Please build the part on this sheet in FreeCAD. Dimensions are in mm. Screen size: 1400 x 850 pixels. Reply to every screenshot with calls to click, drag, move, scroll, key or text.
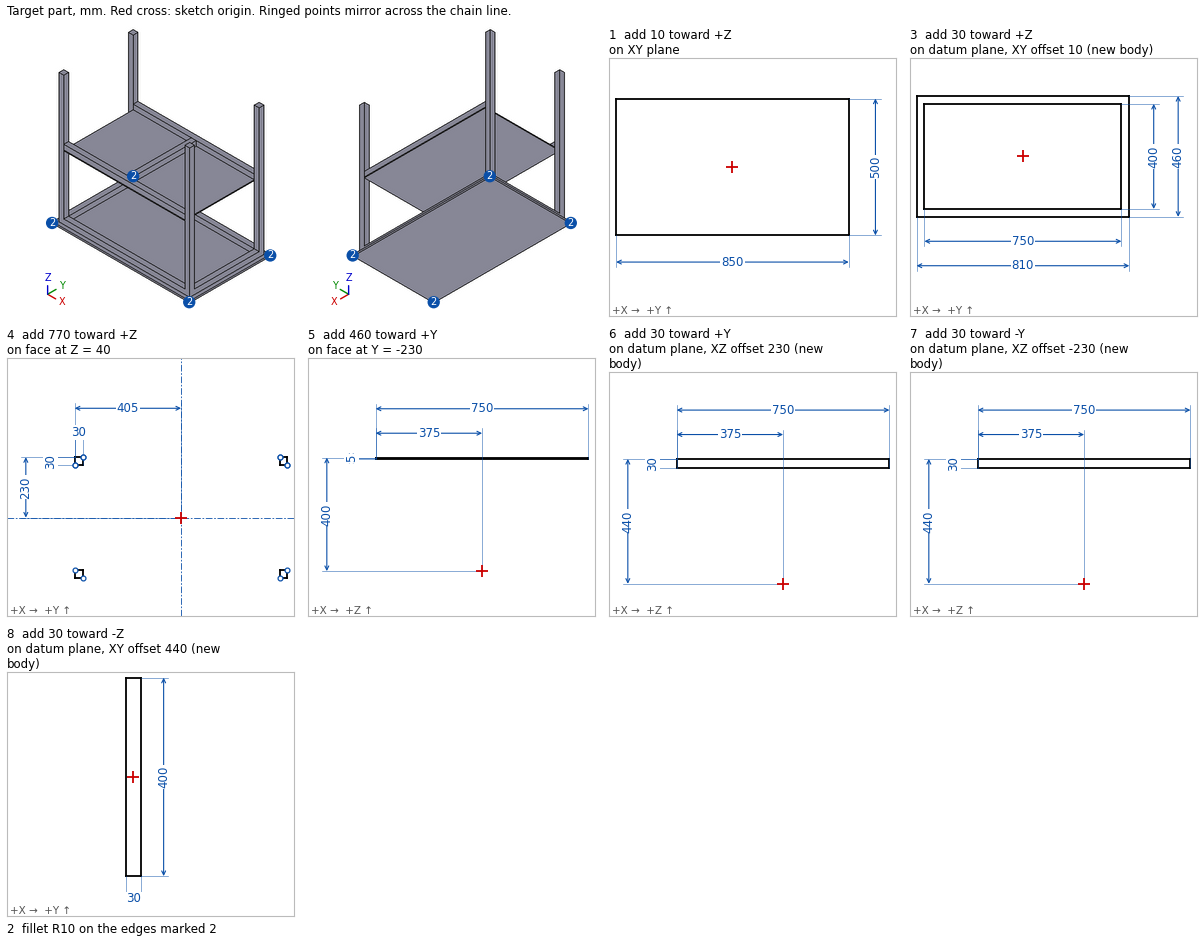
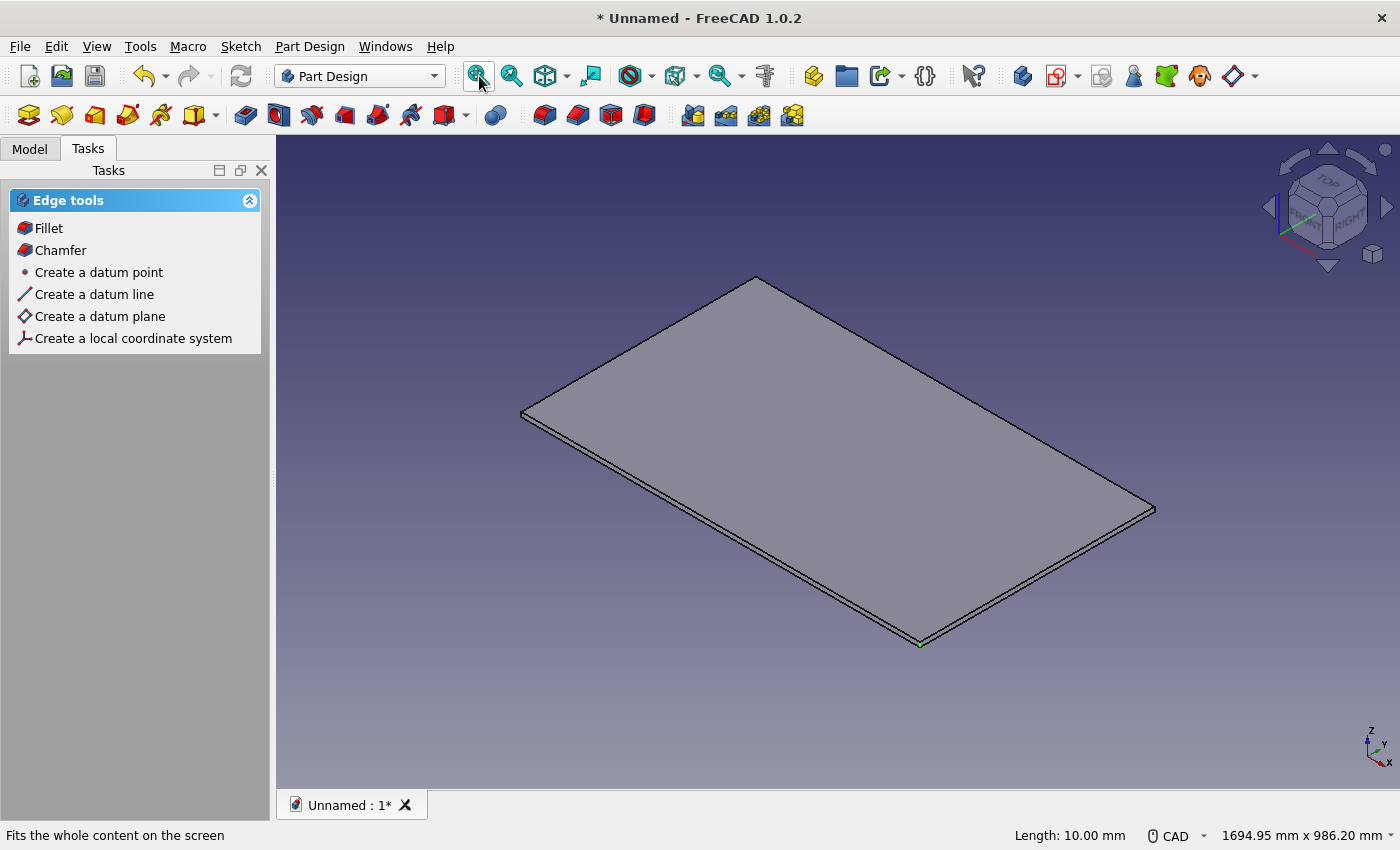
scroll(521, 414, up, 9)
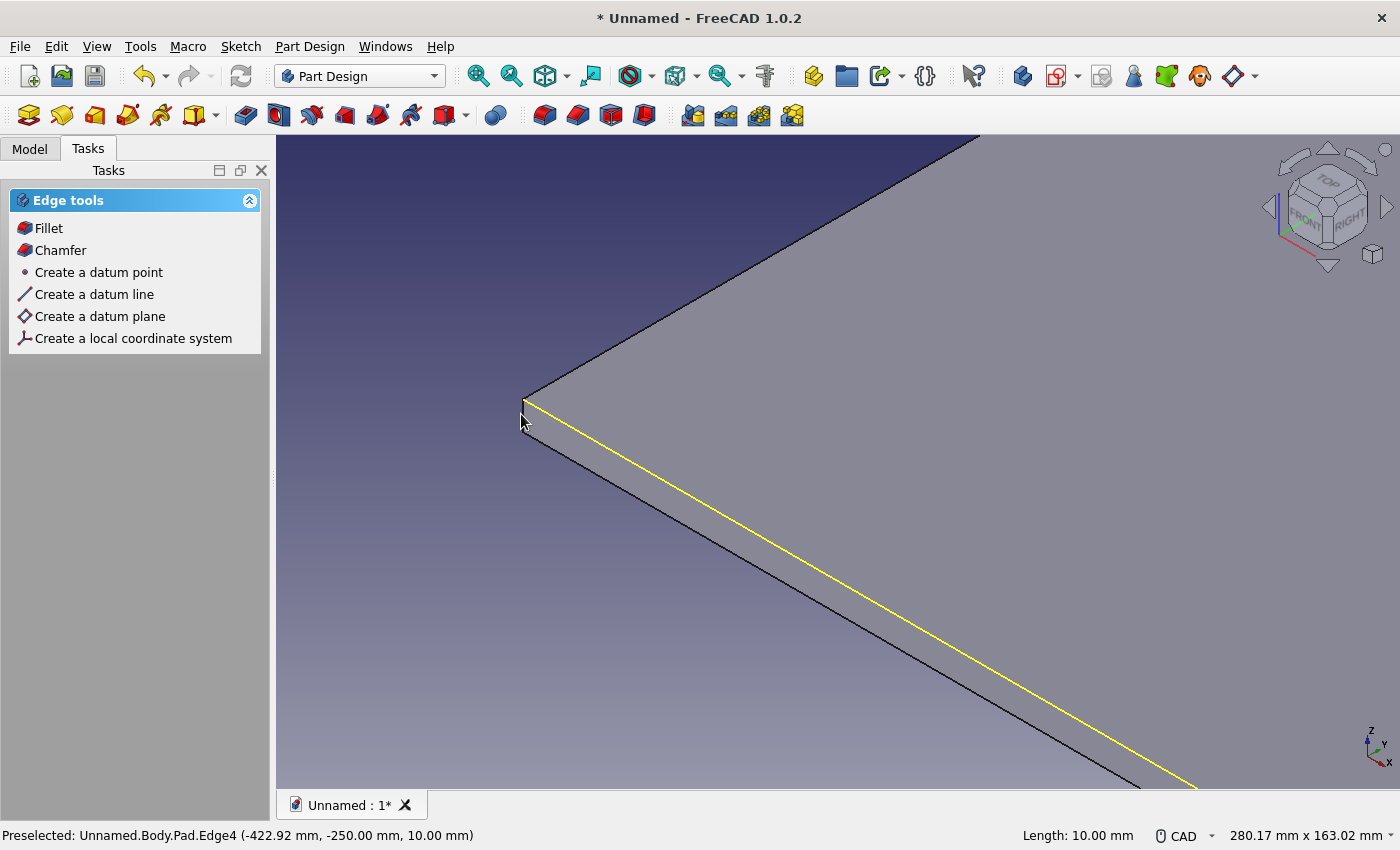
click(479, 76)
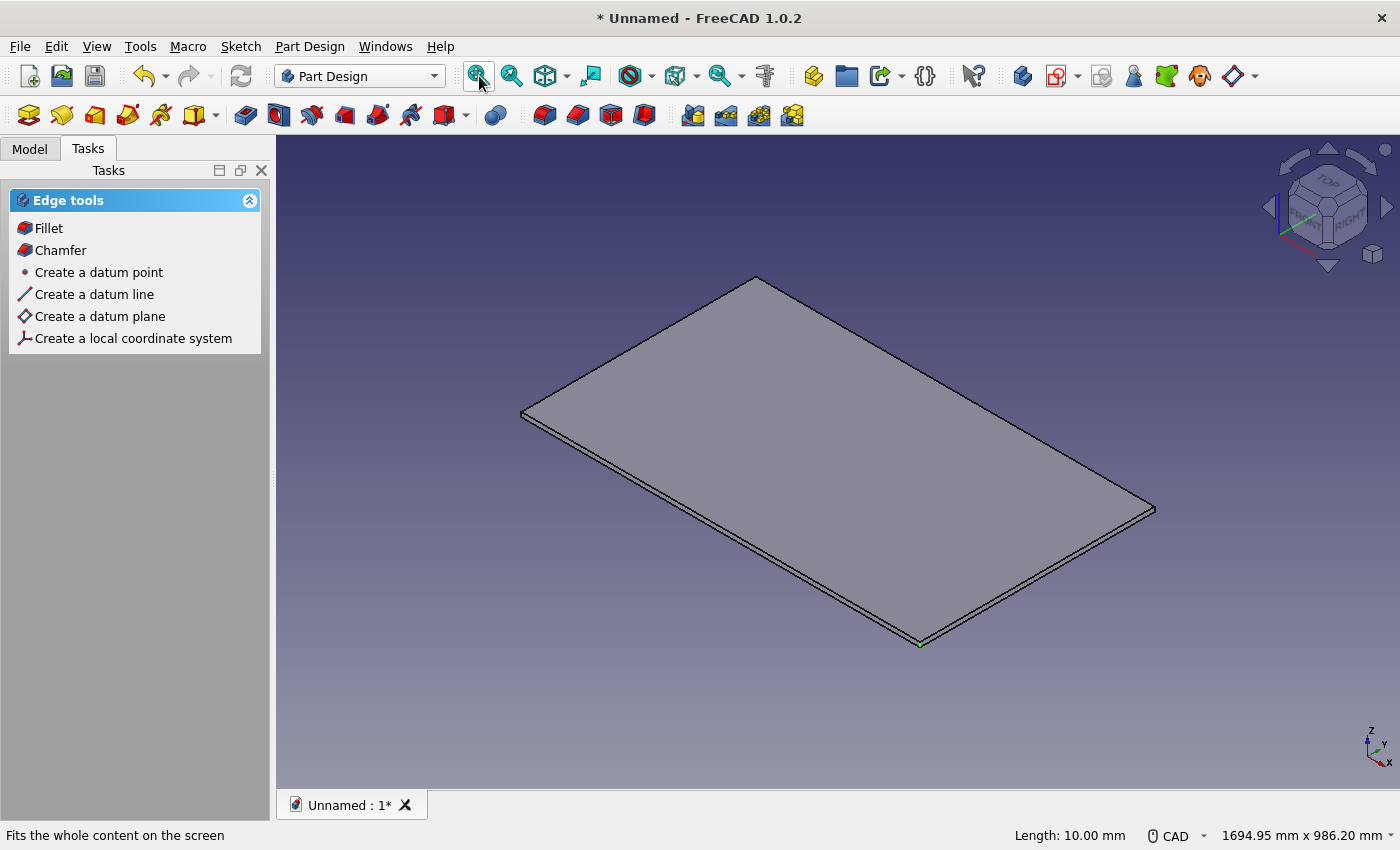
key(2)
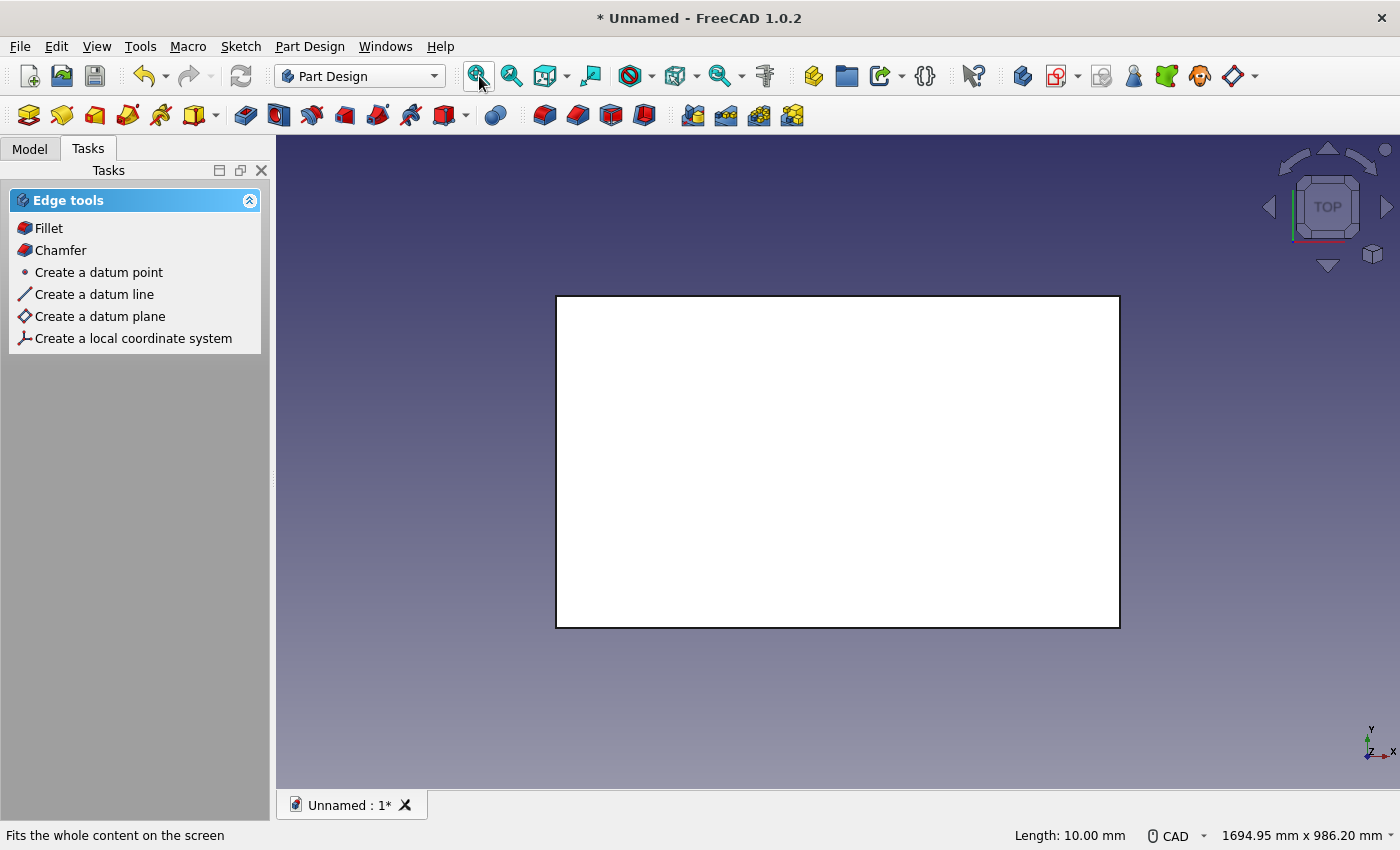
scroll(556, 627, up, 9)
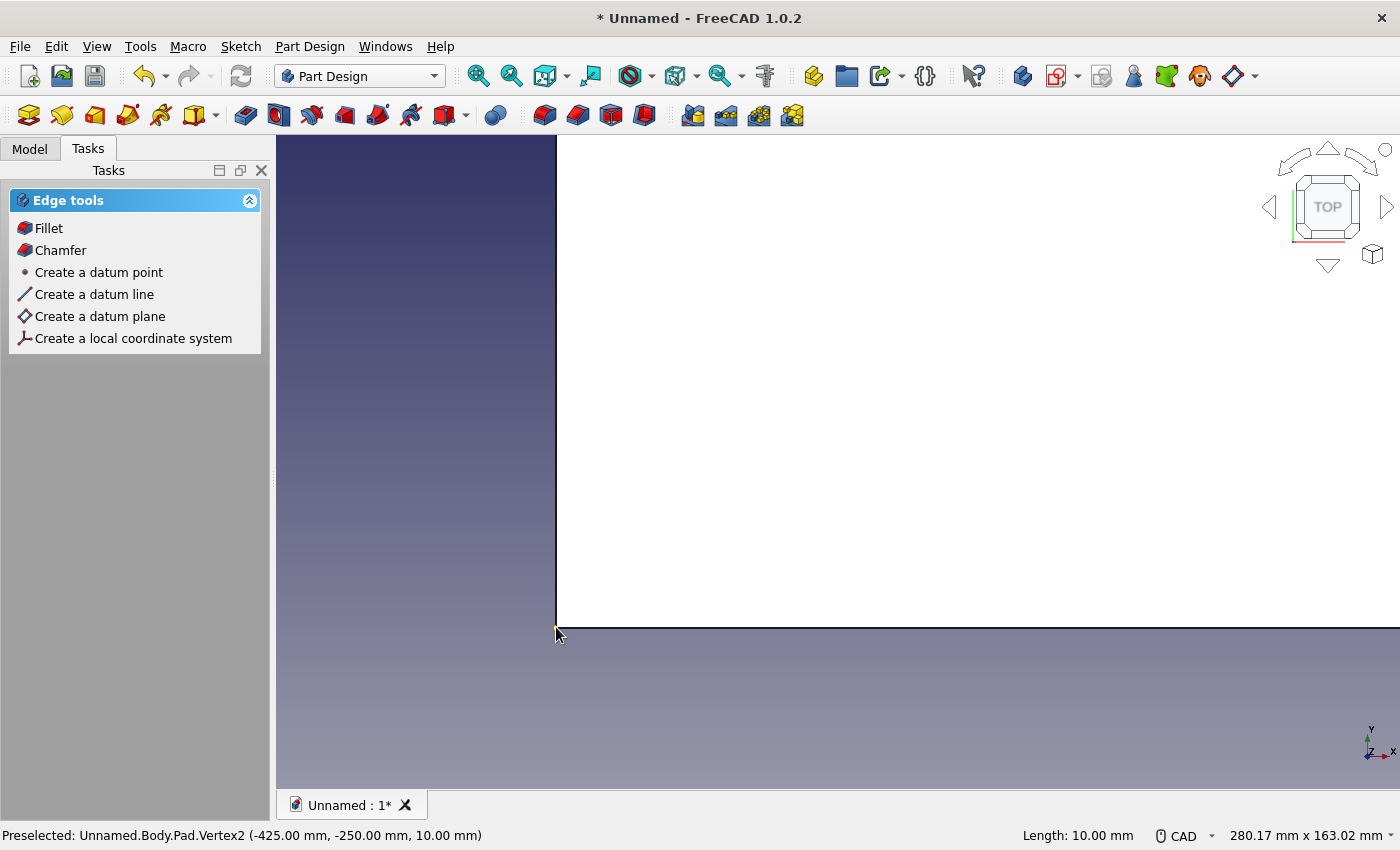
click(479, 76)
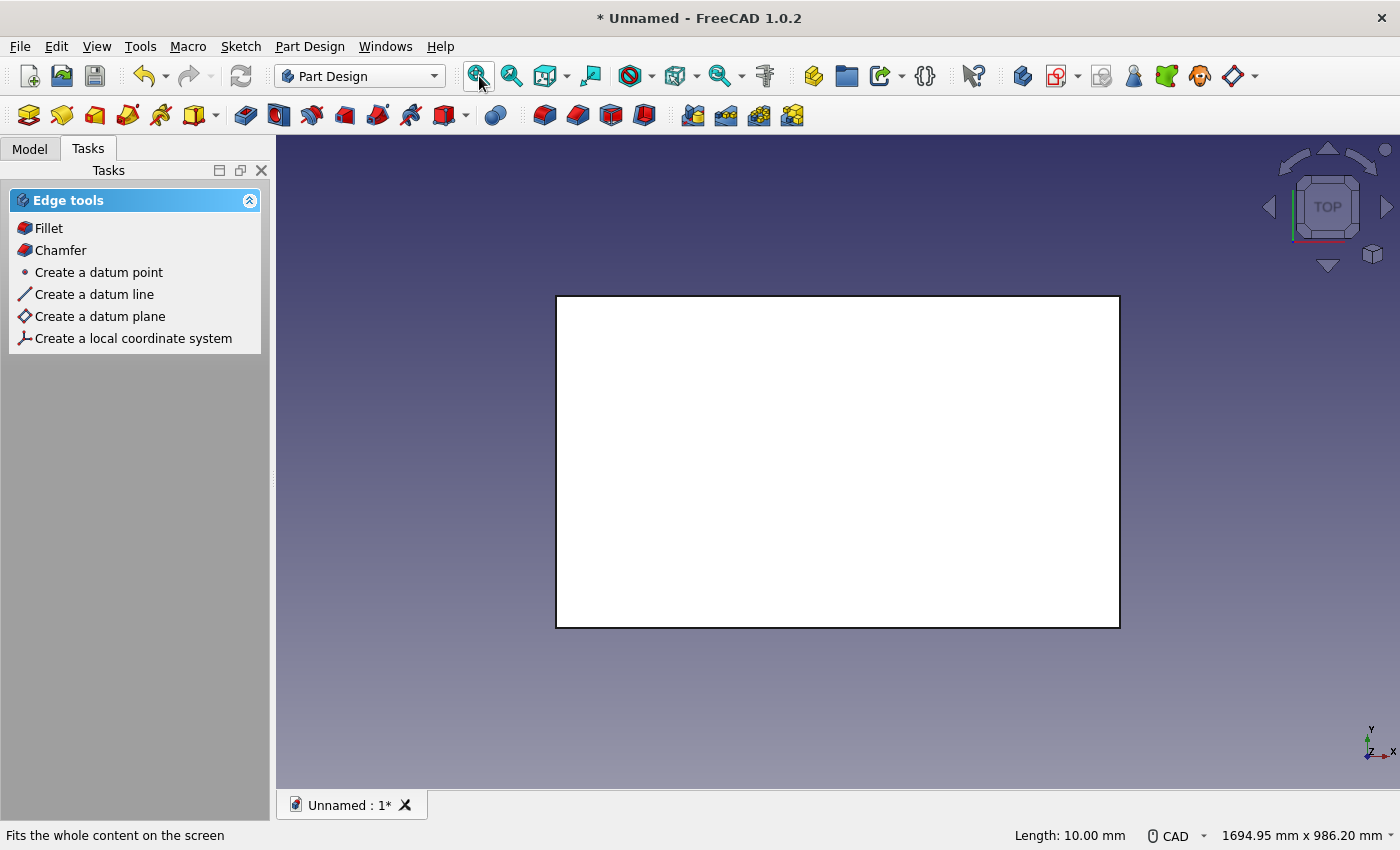
key(1)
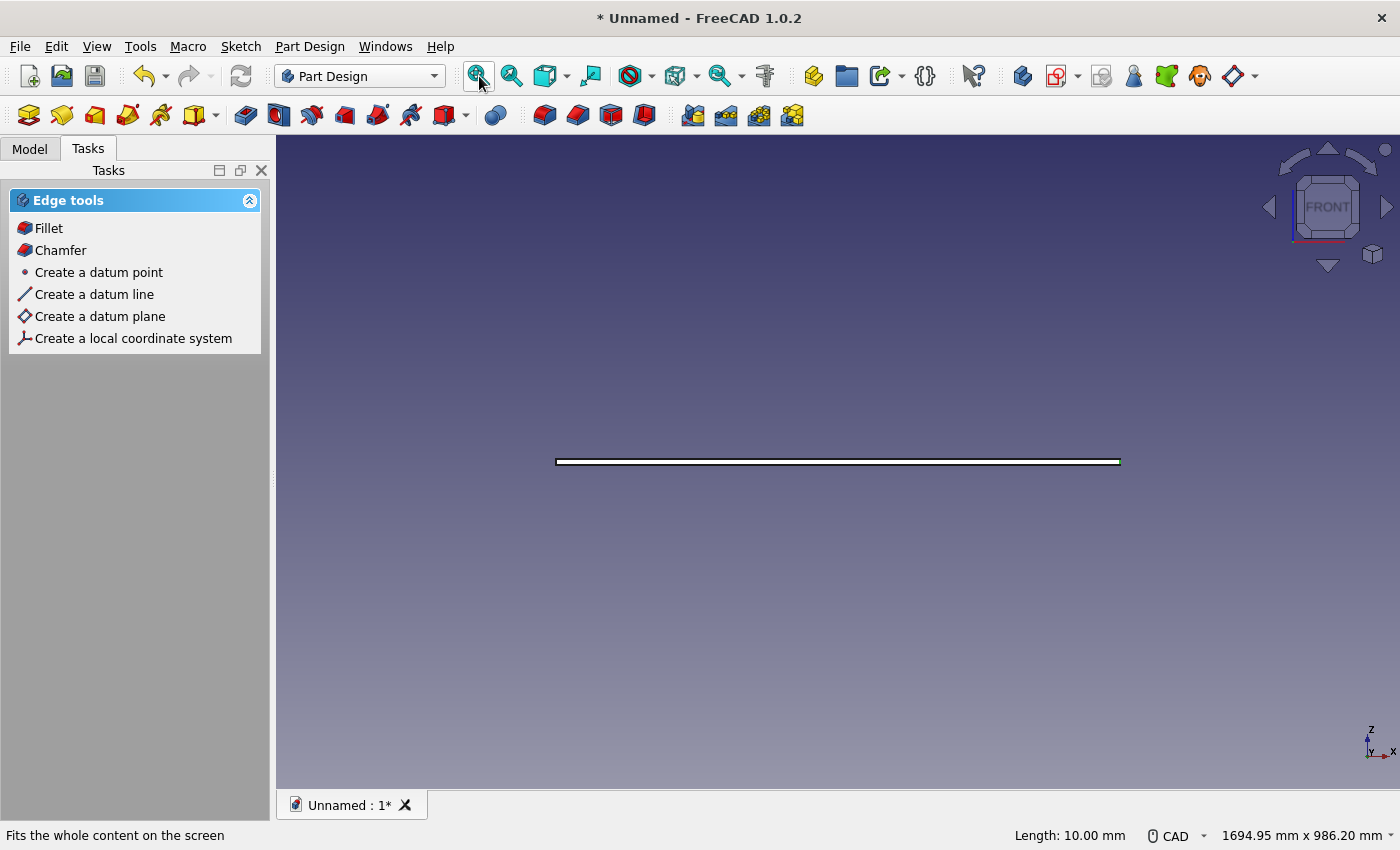
scroll(556, 461, up, 9)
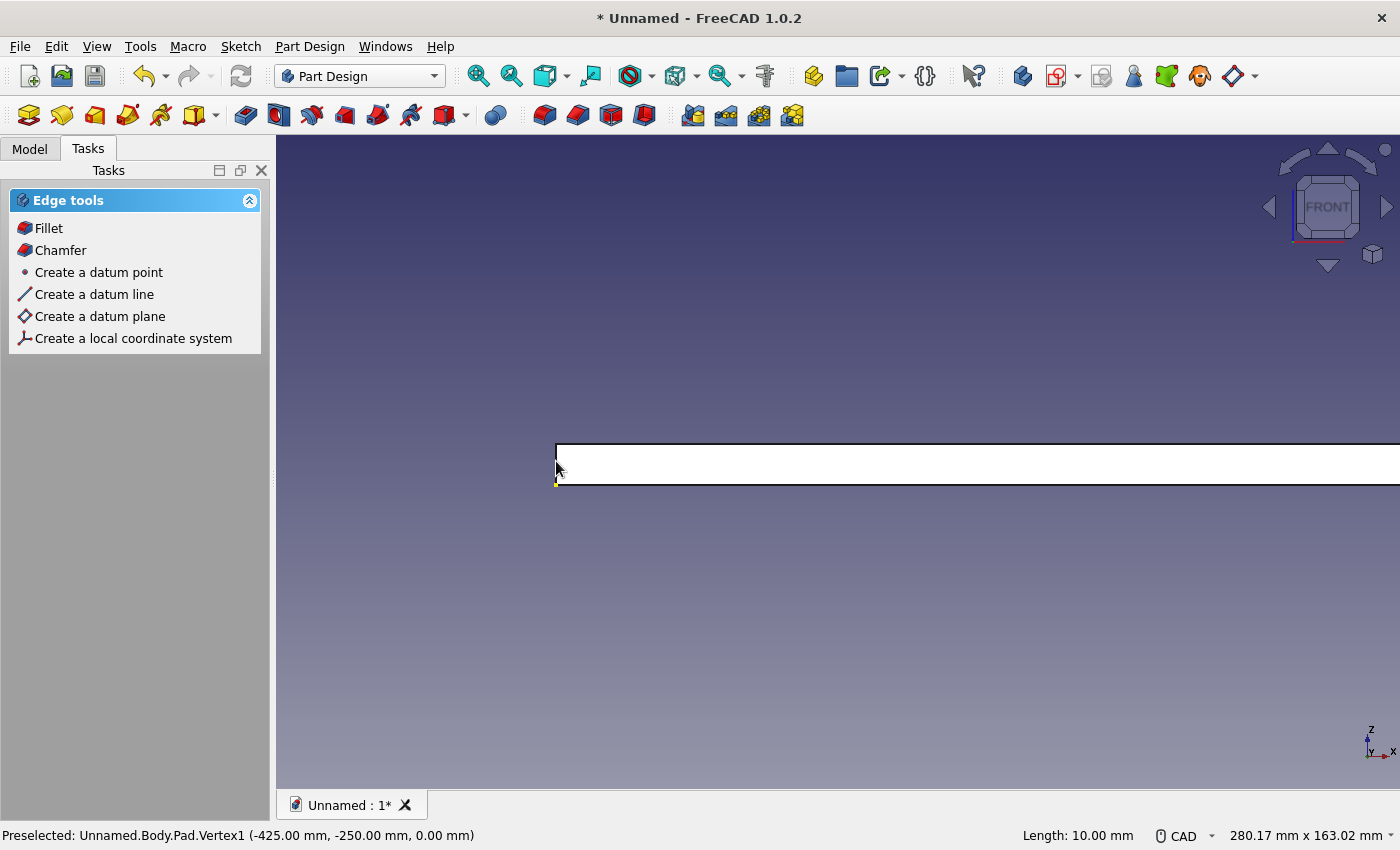
click(556, 464, ctrl)